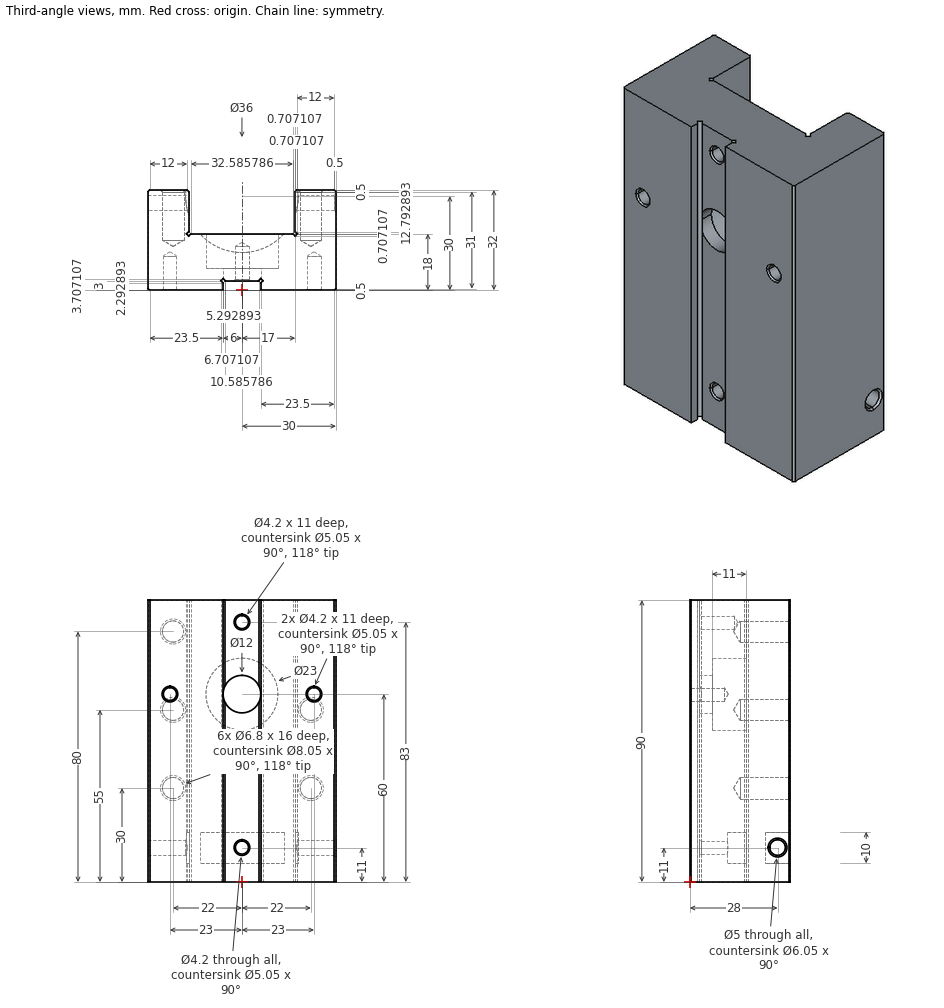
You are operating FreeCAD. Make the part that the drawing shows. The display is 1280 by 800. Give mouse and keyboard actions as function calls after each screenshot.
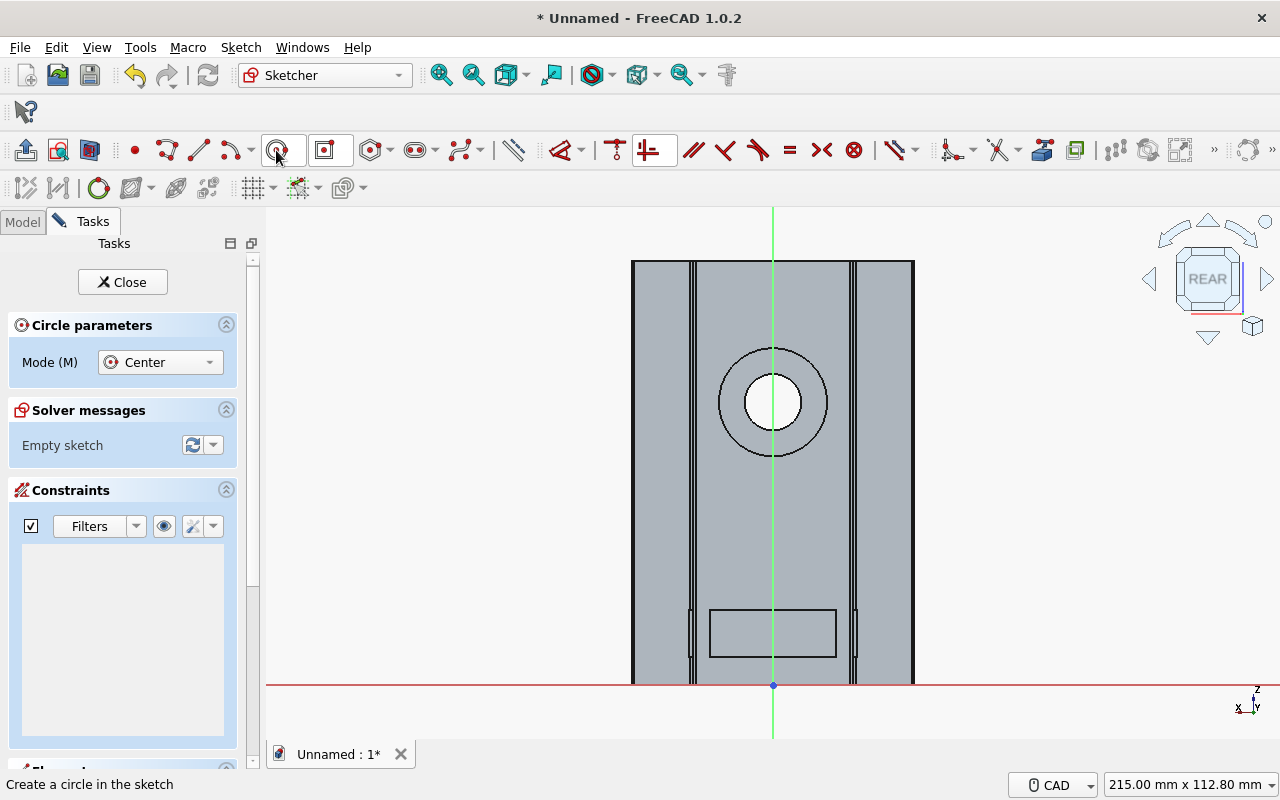
scroll(877, 544, up, 2)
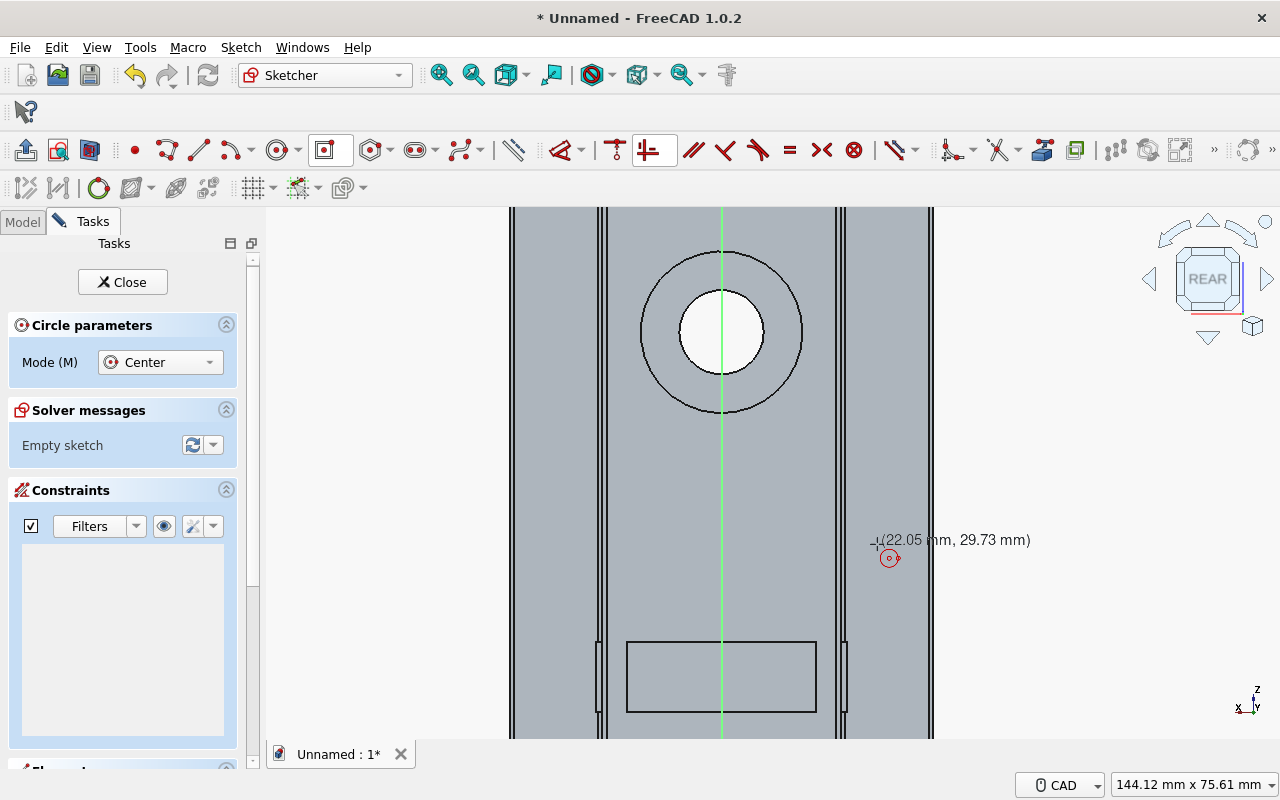
click(876, 543)
move(893, 526)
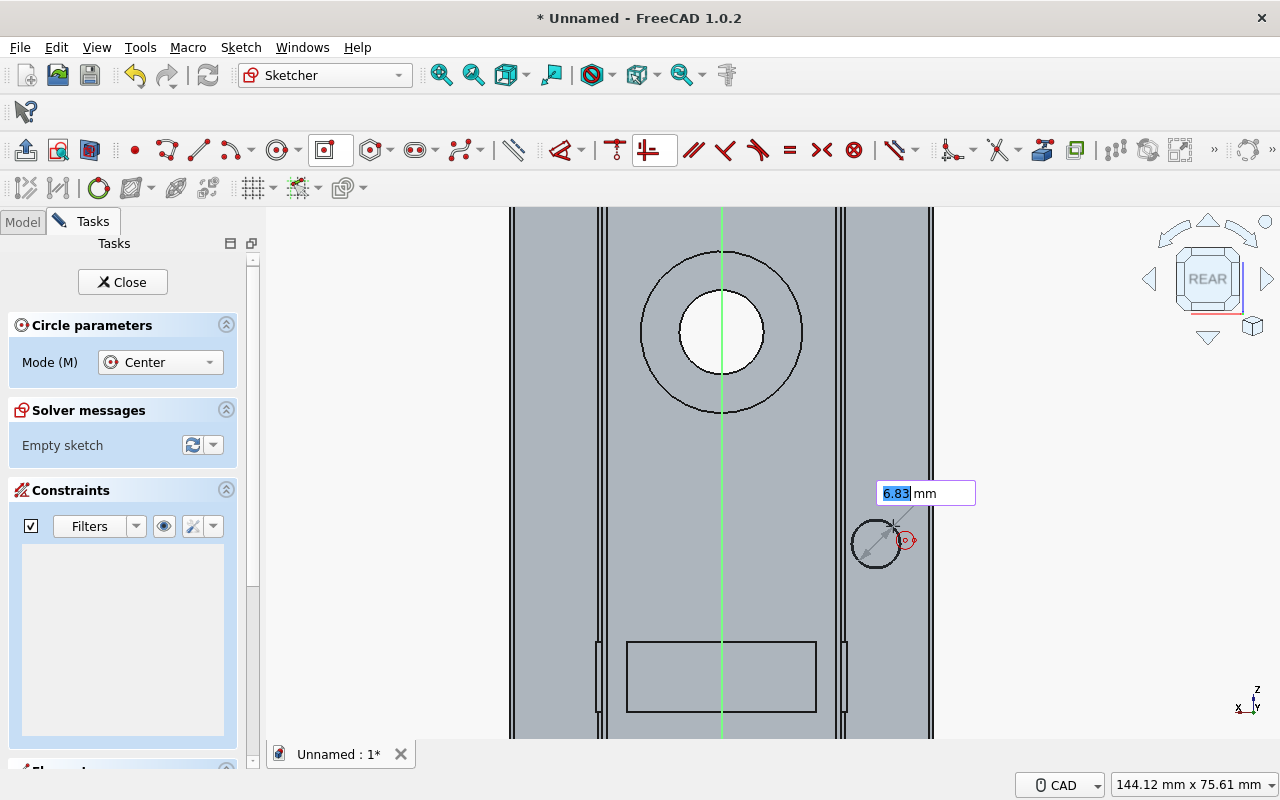
text(6.8)
key(Return)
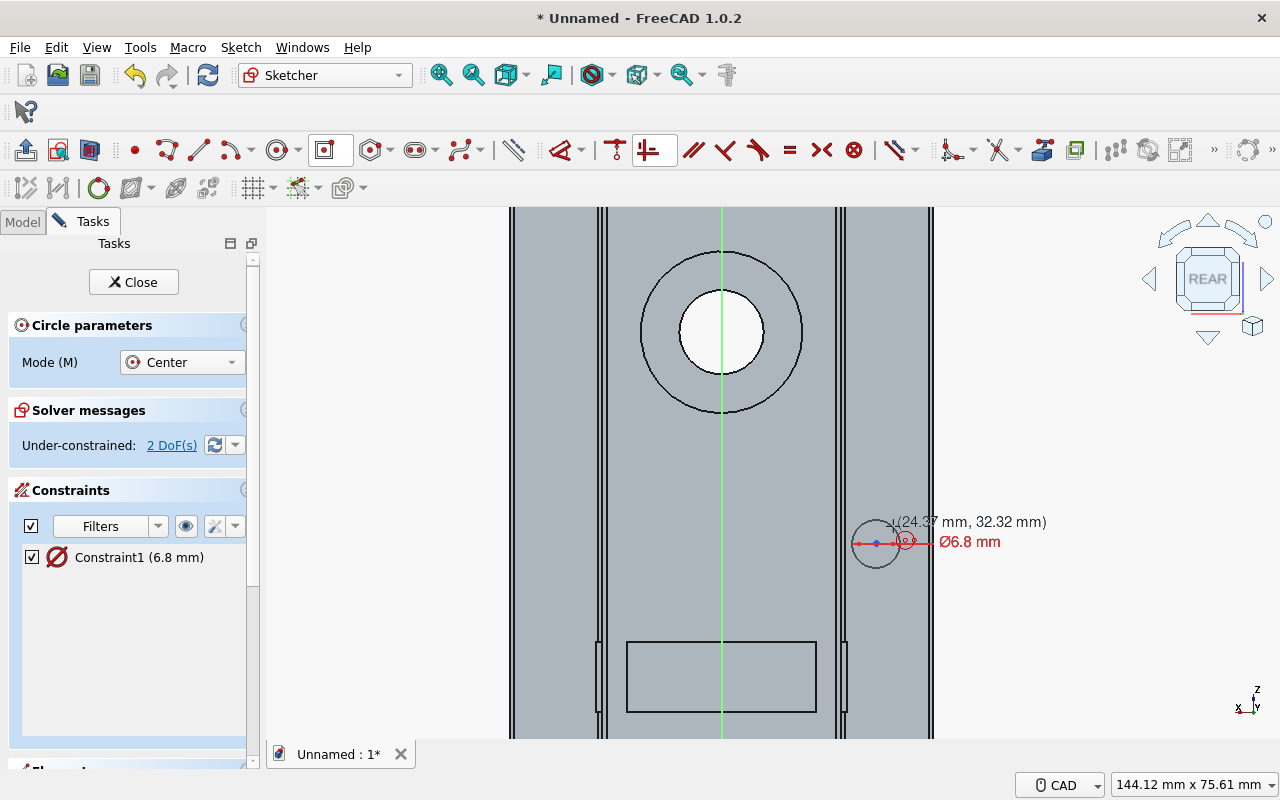
click(876, 367)
move(893, 350)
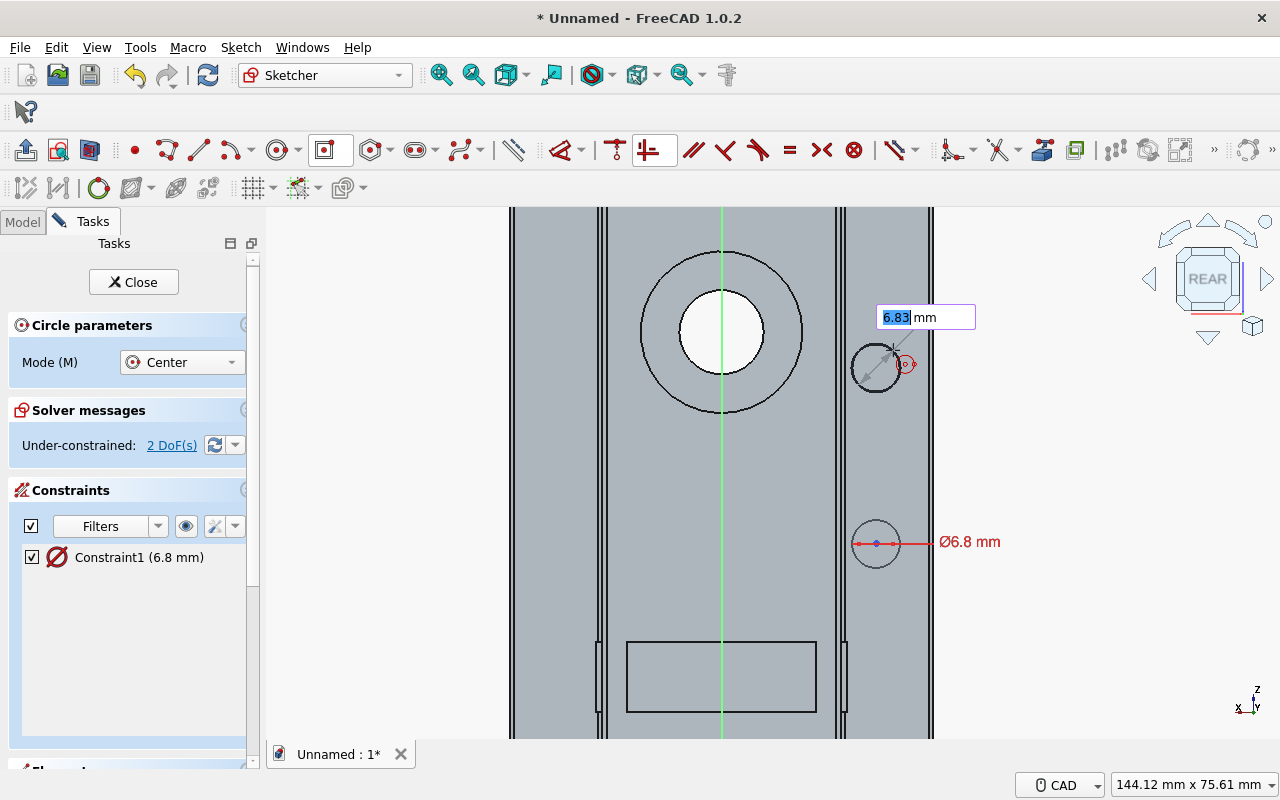
text(6.8)
key(Return)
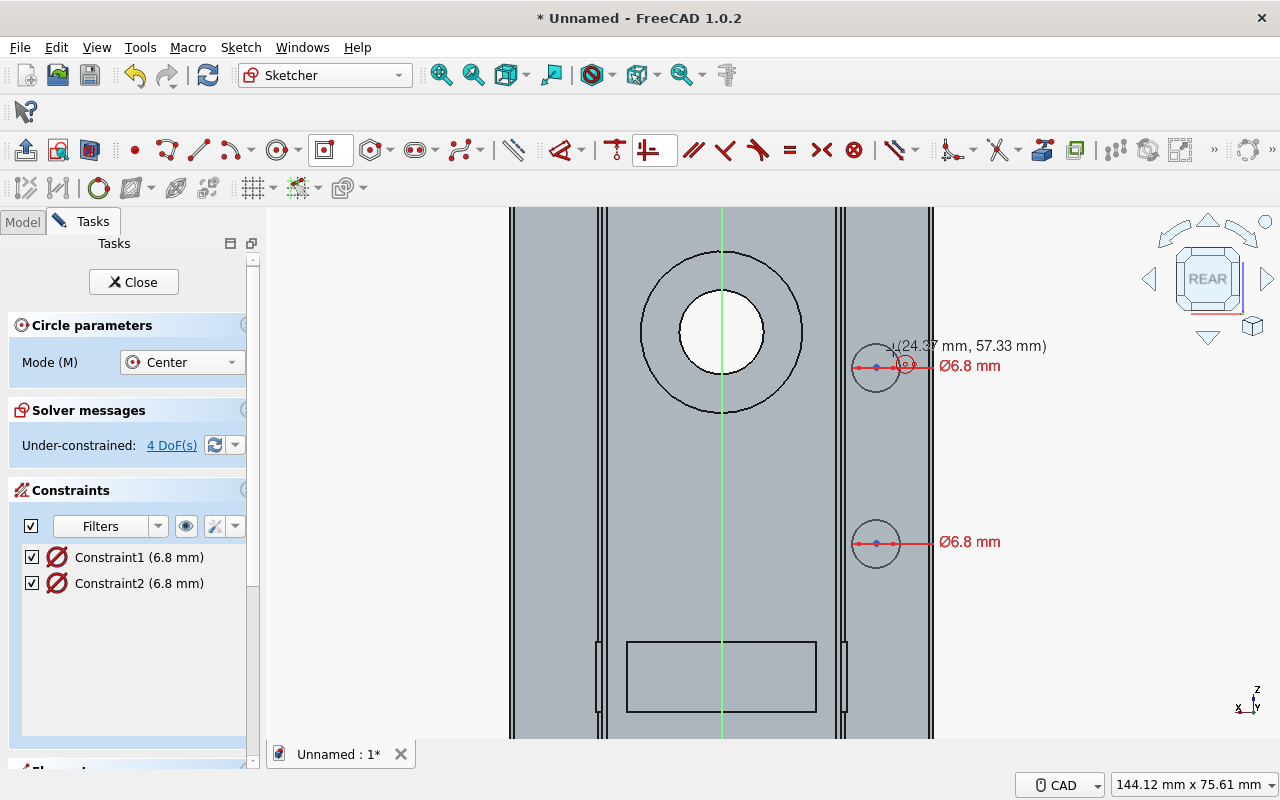
scroll(684, 488, down, 3)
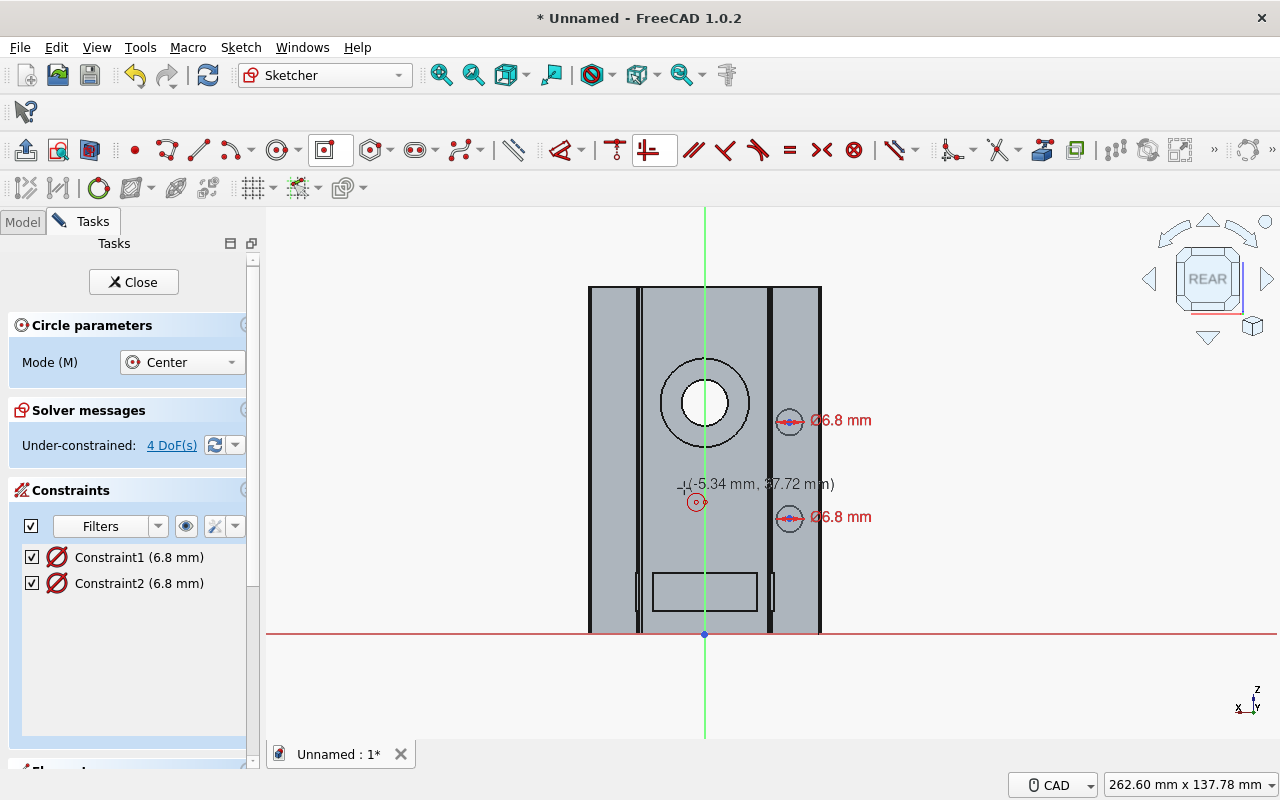
scroll(790, 326, up, 3)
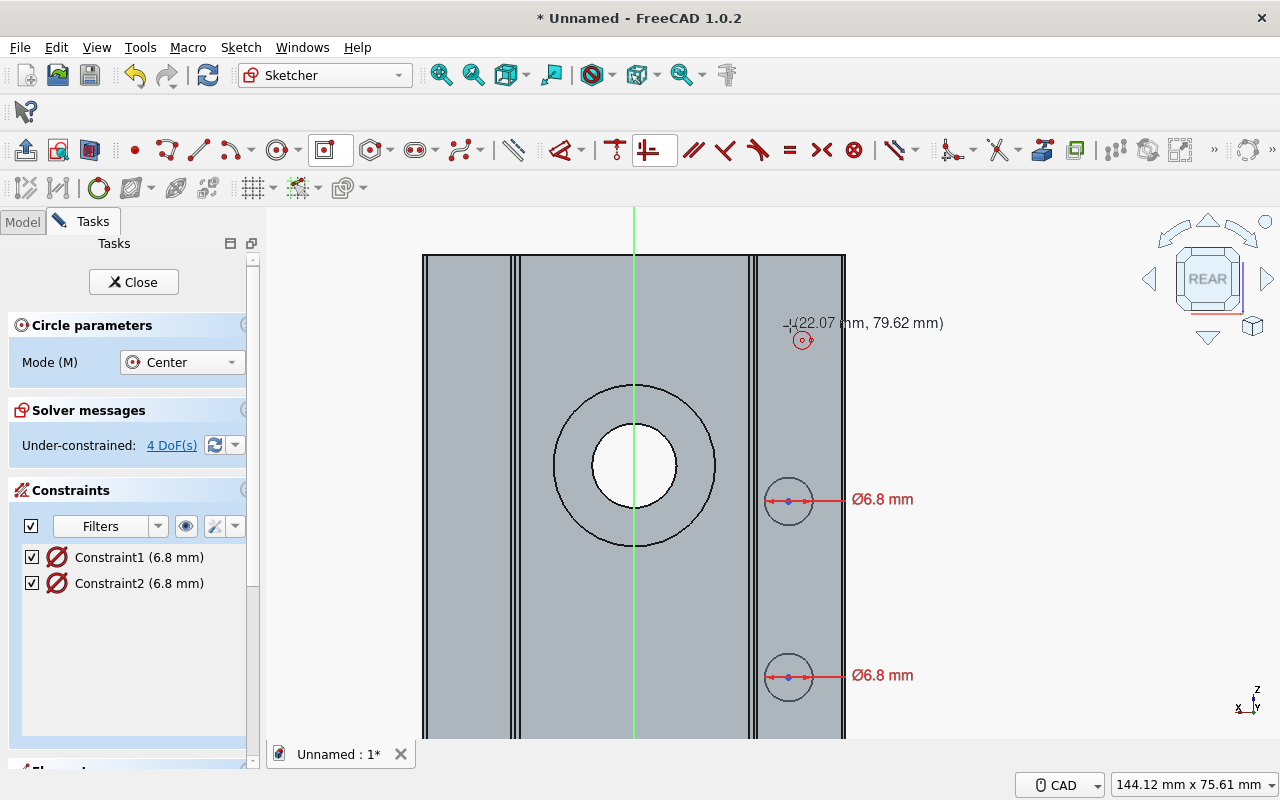
click(789, 325)
move(806, 308)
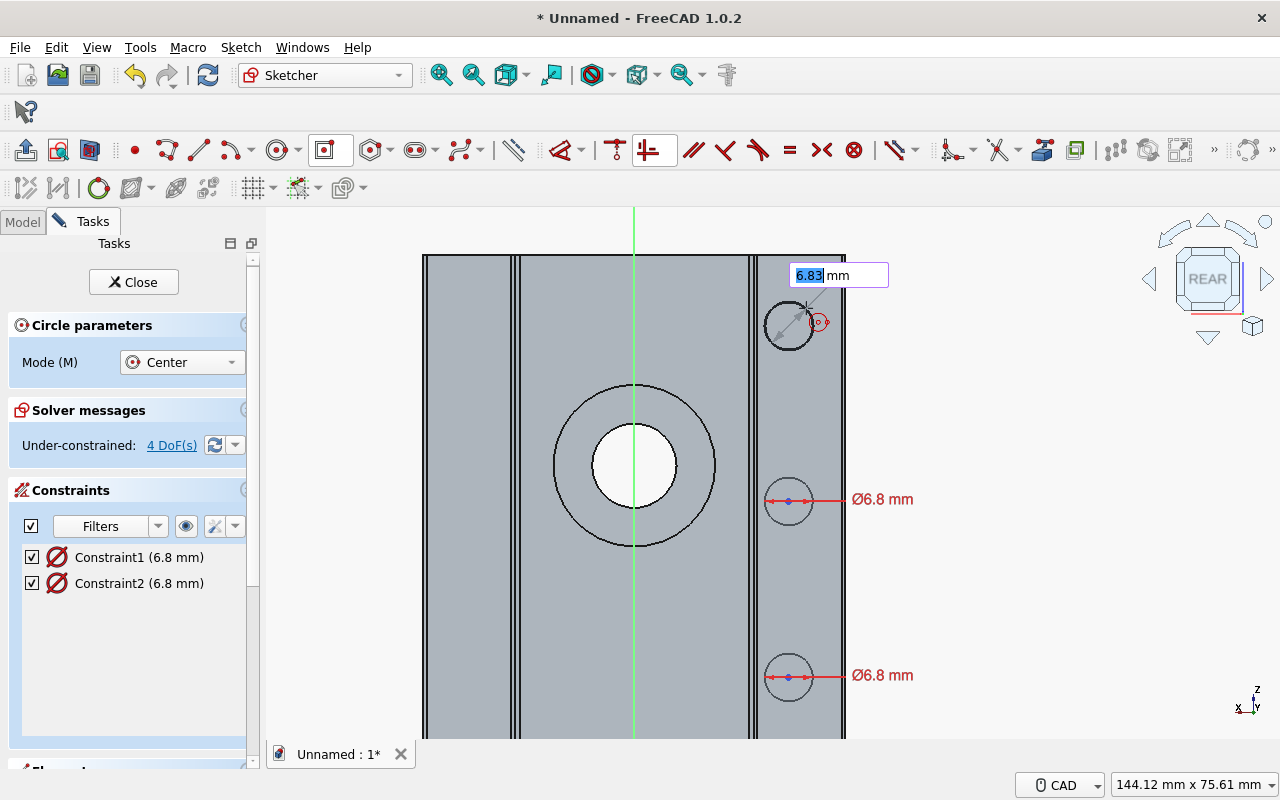
text(6.8)
key(Return)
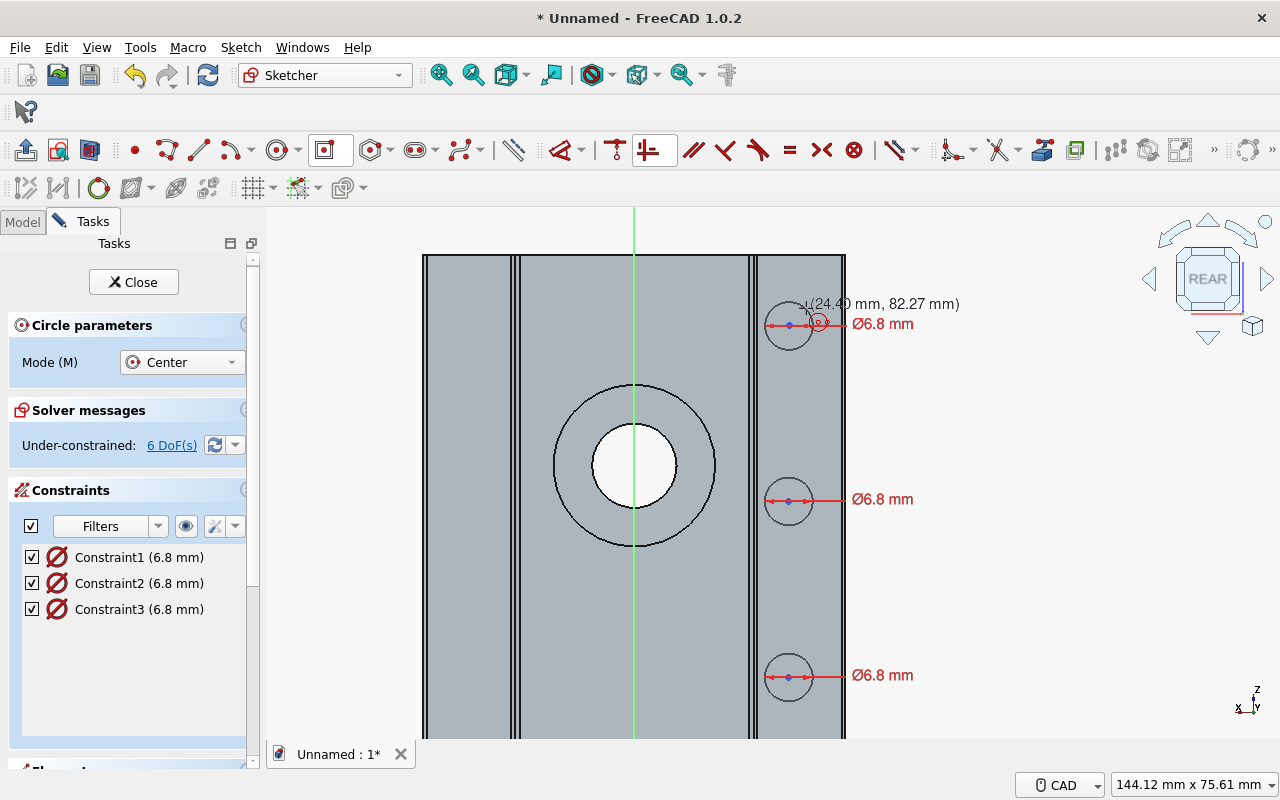
click(480, 677)
move(496, 660)